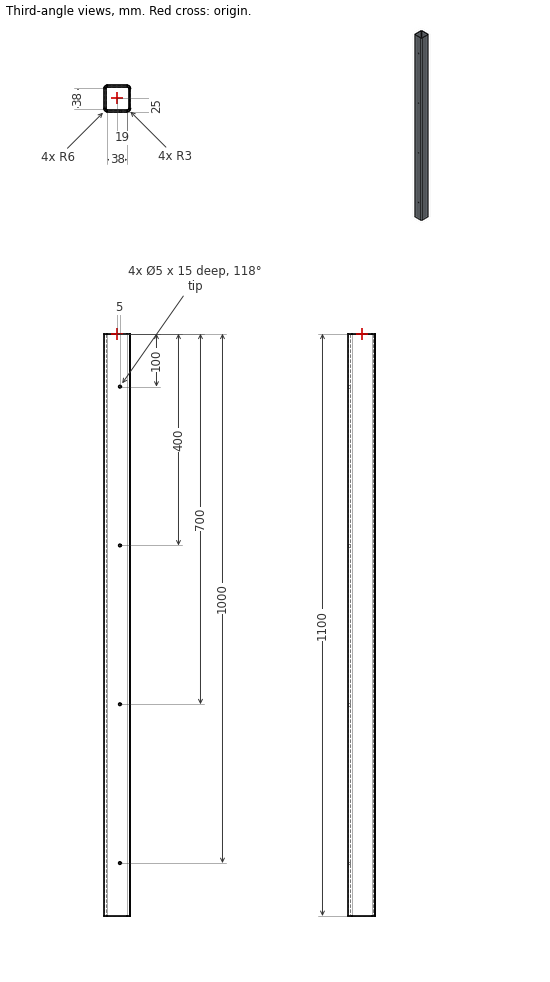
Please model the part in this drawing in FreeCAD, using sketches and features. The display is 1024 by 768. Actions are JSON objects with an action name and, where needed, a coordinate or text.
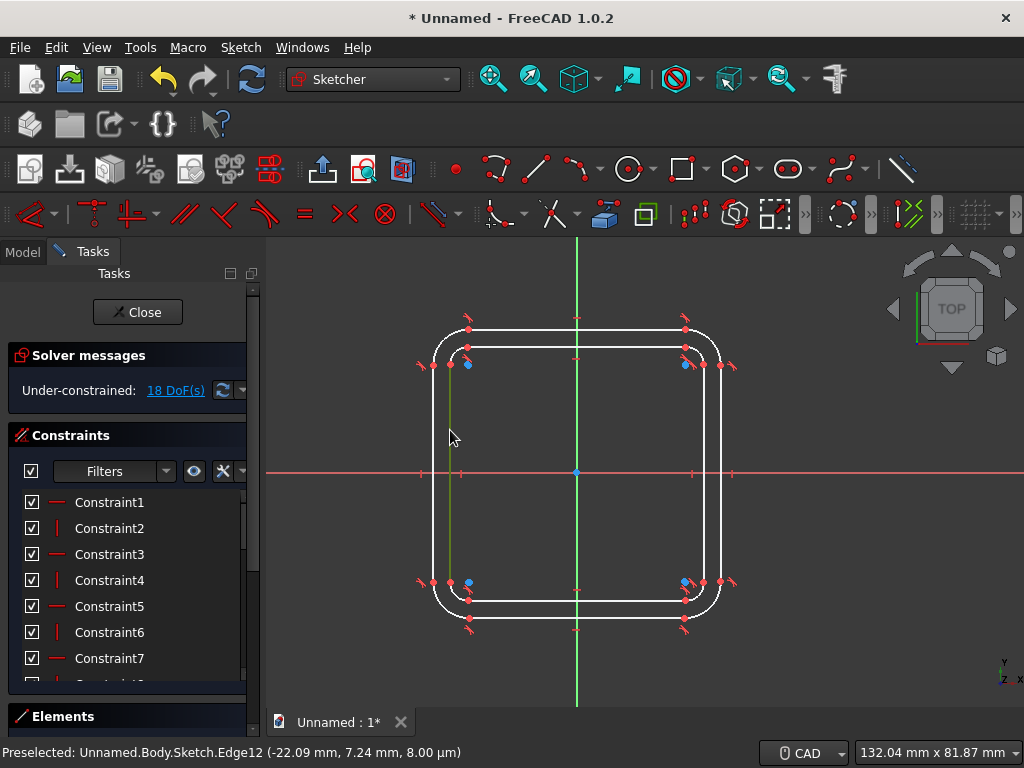
{"action": "left_click", "coordinate": [455, 352]}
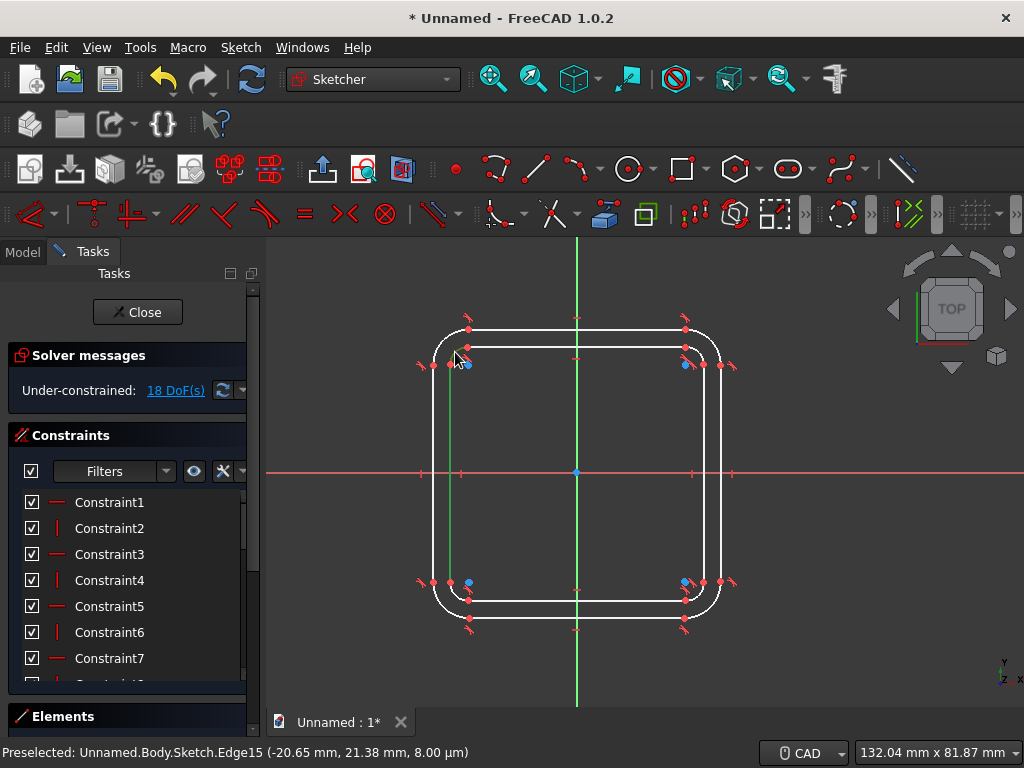
{"action": "key", "text": "t"}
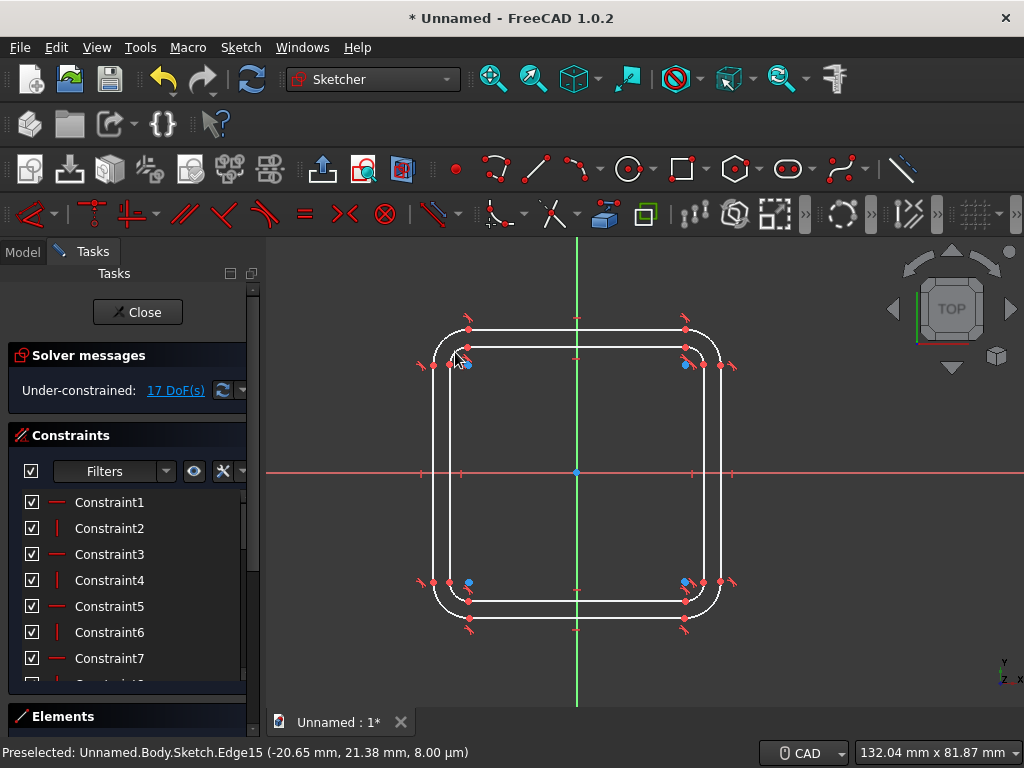
{"action": "left_click", "coordinate": [450, 430]}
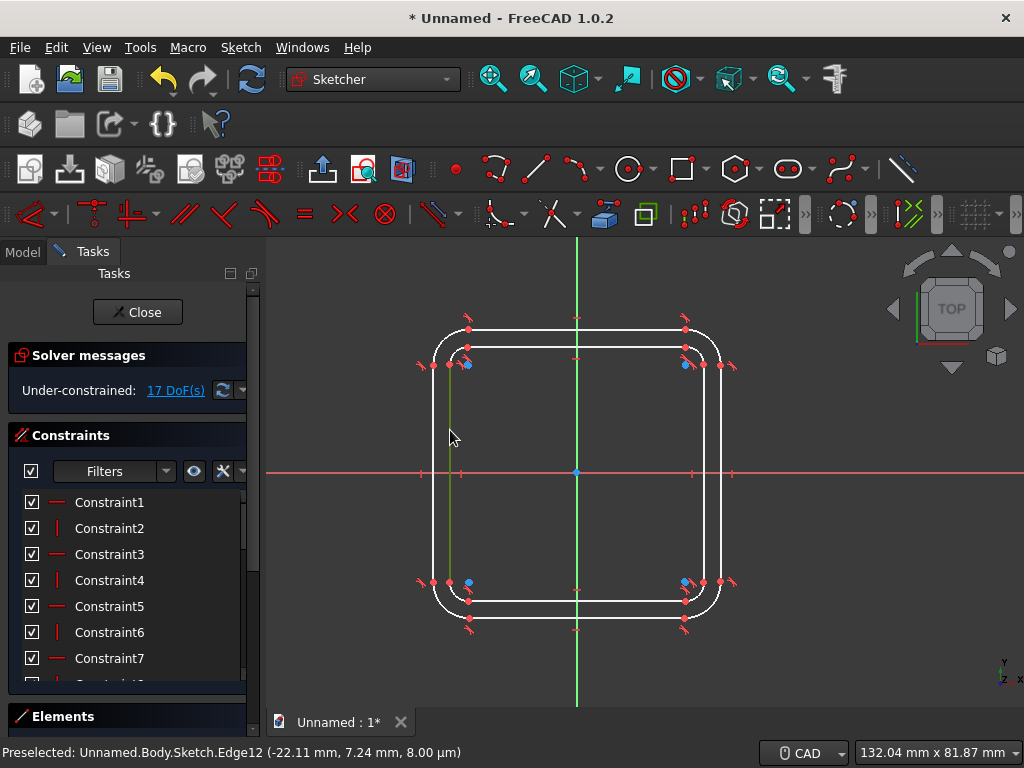
{"action": "left_click", "coordinate": [456, 596]}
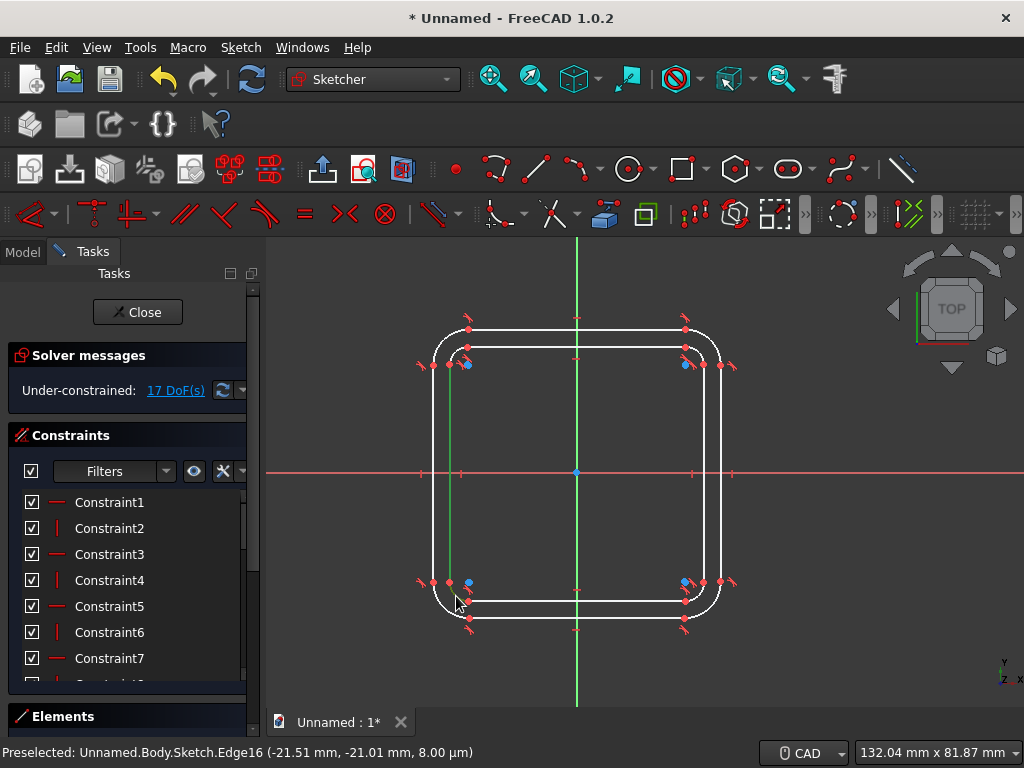
{"action": "key", "text": "t"}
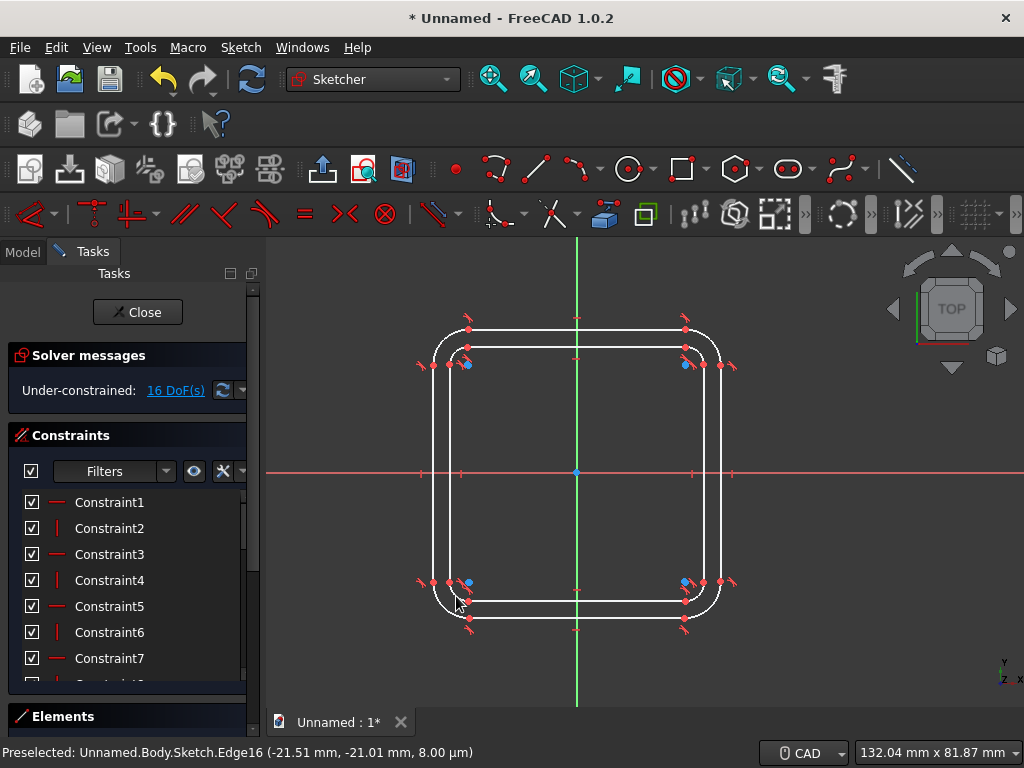
{"action": "left_click", "coordinate": [701, 614]}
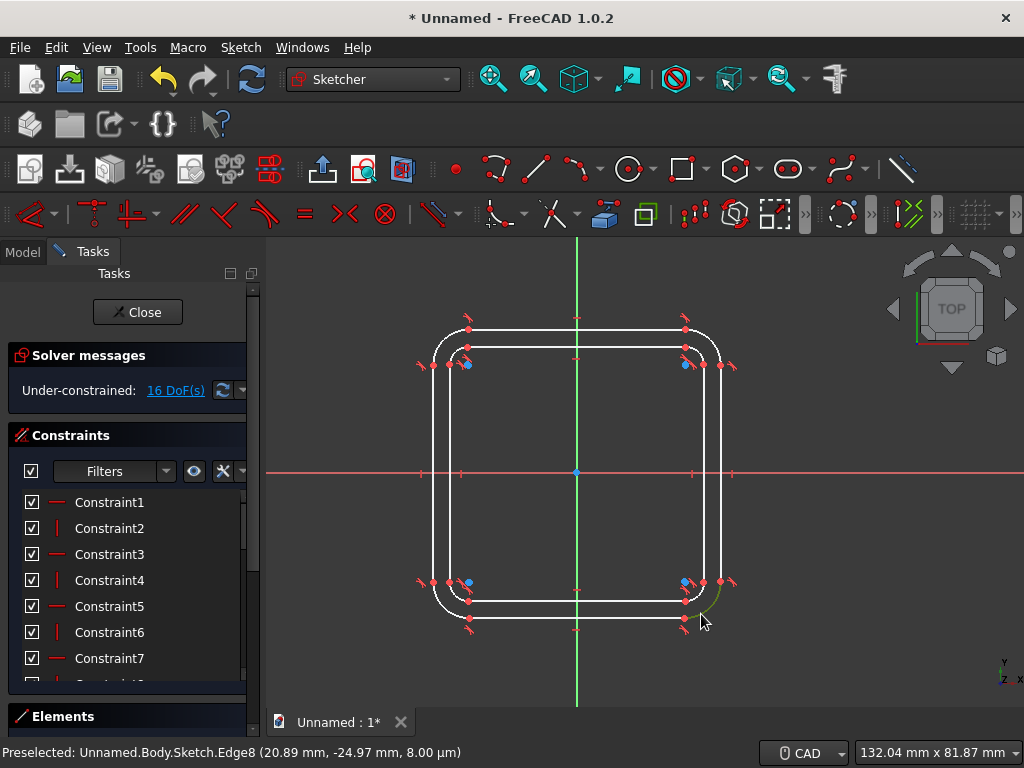
{"action": "left_click", "coordinate": [699, 596]}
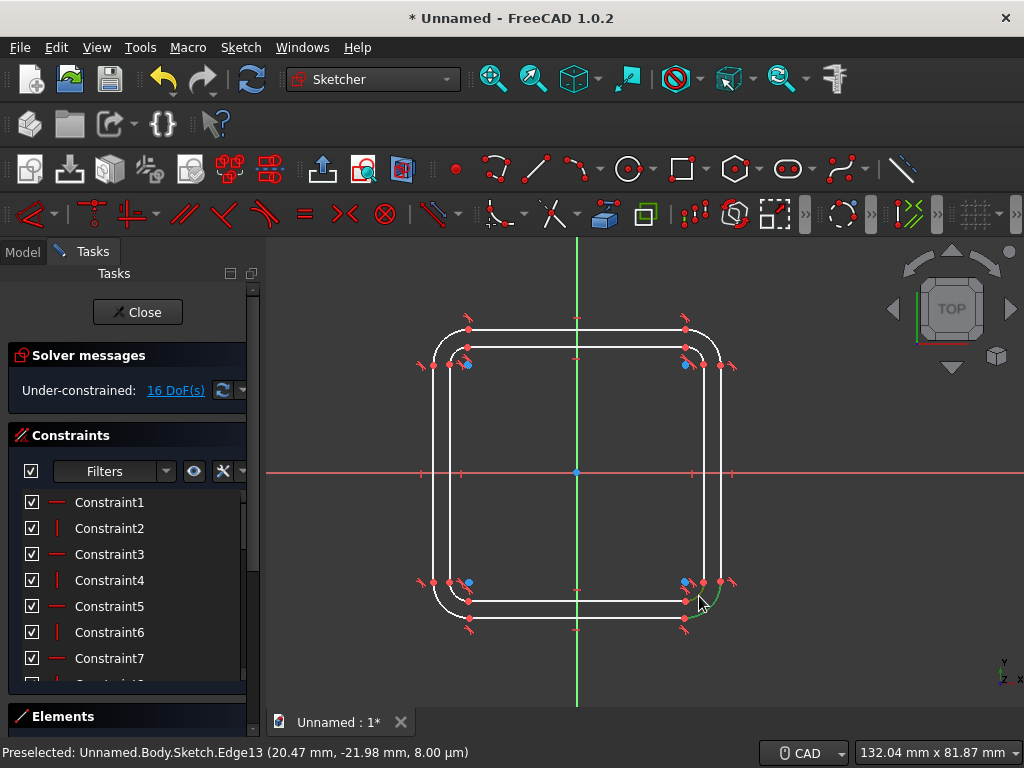
{"action": "key", "text": "c"}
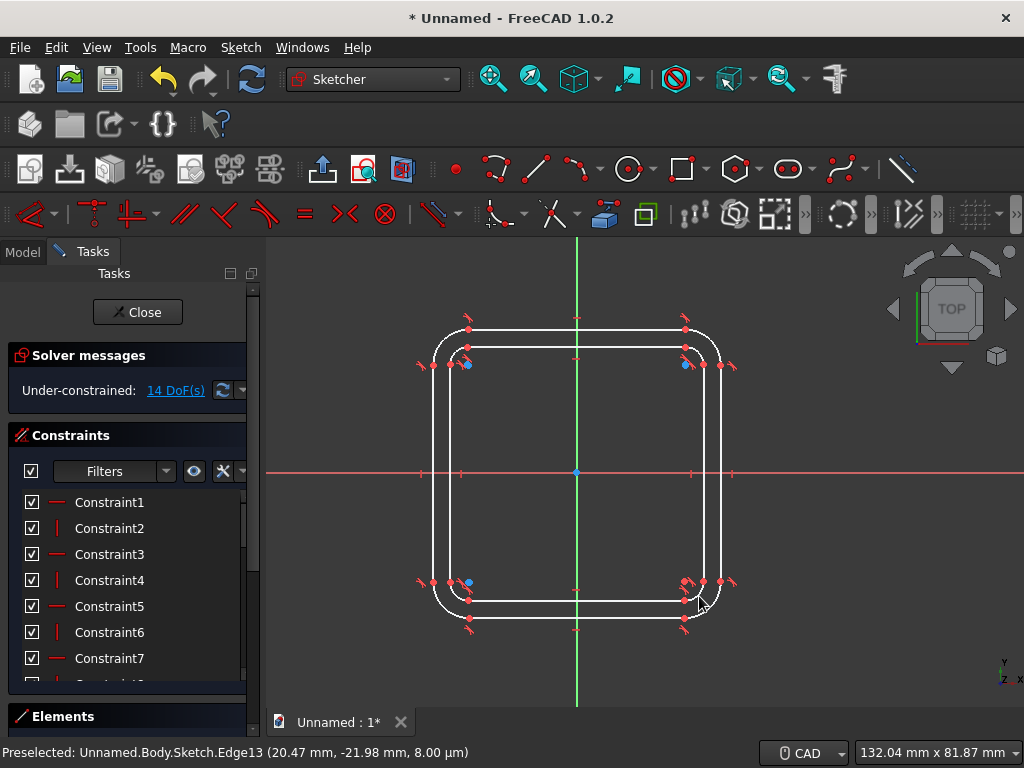
{"action": "left_click", "coordinate": [717, 349]}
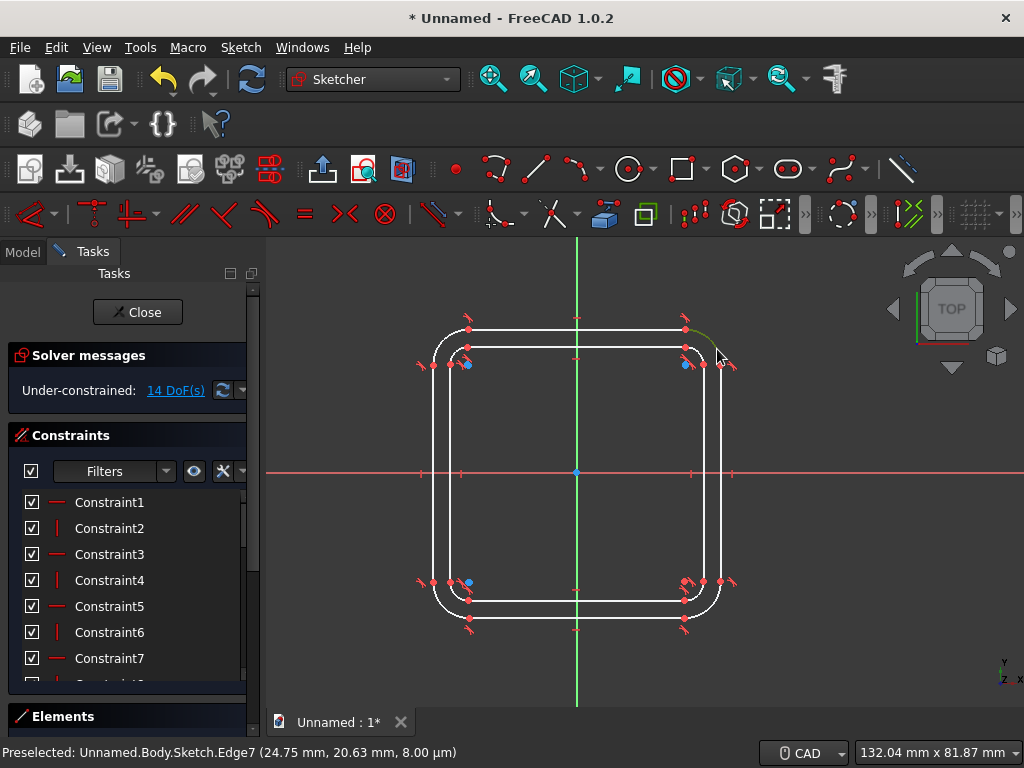
{"action": "left_click", "coordinate": [698, 352]}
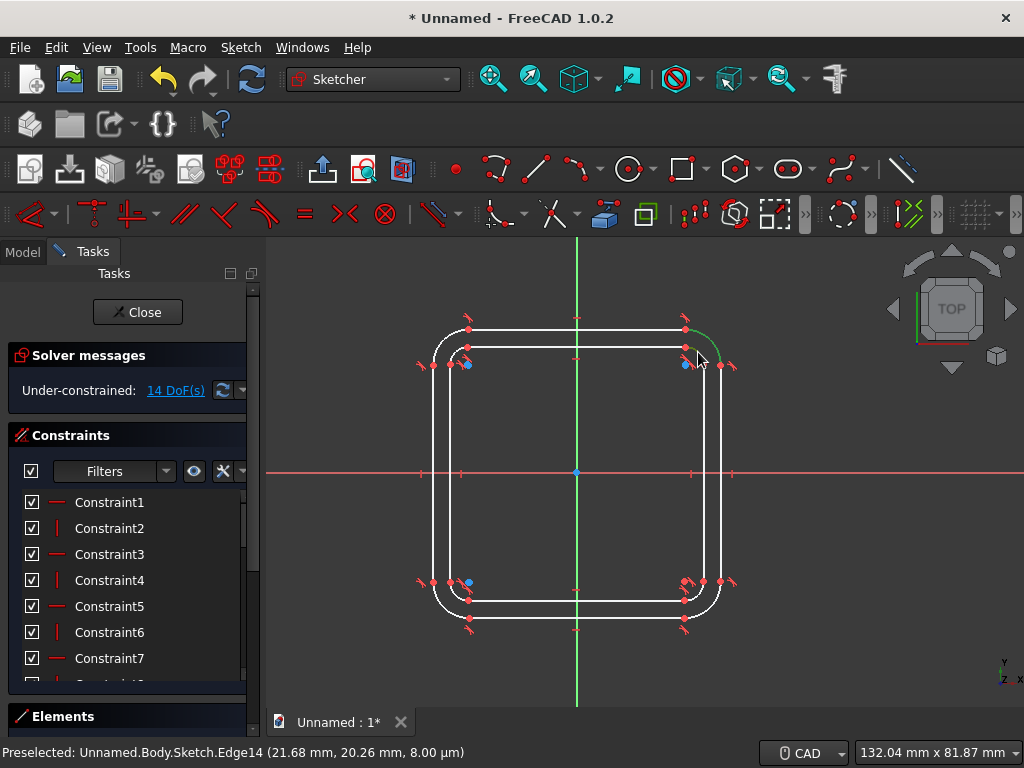
{"action": "key", "text": "c"}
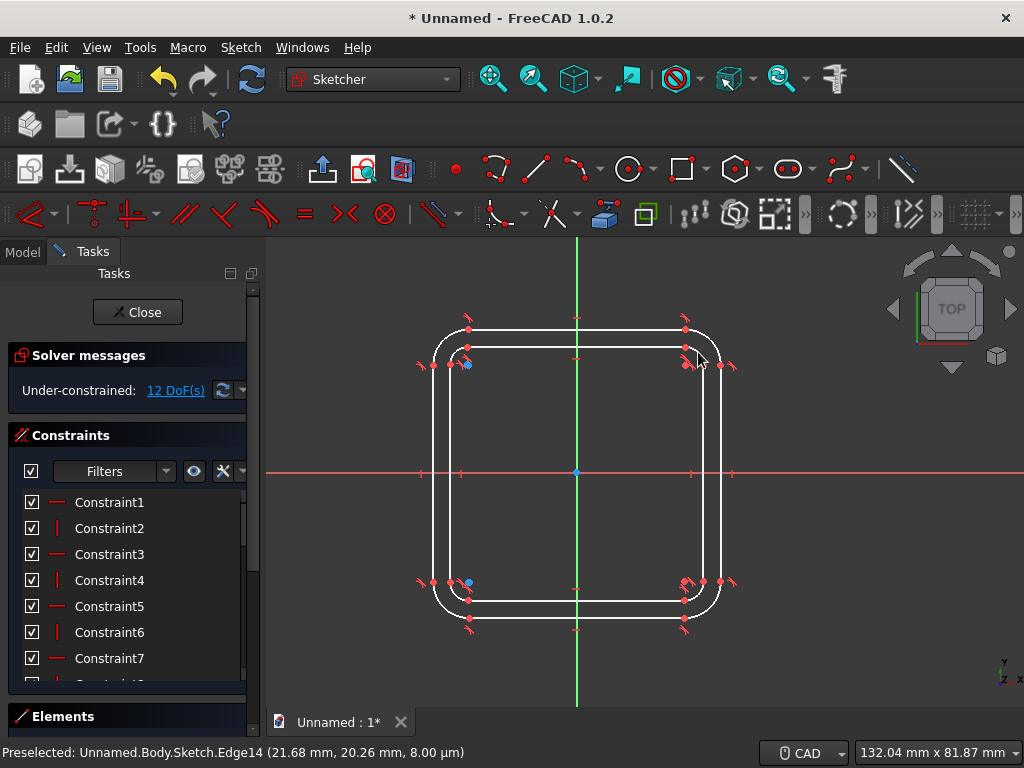
{"action": "left_click", "coordinate": [453, 334]}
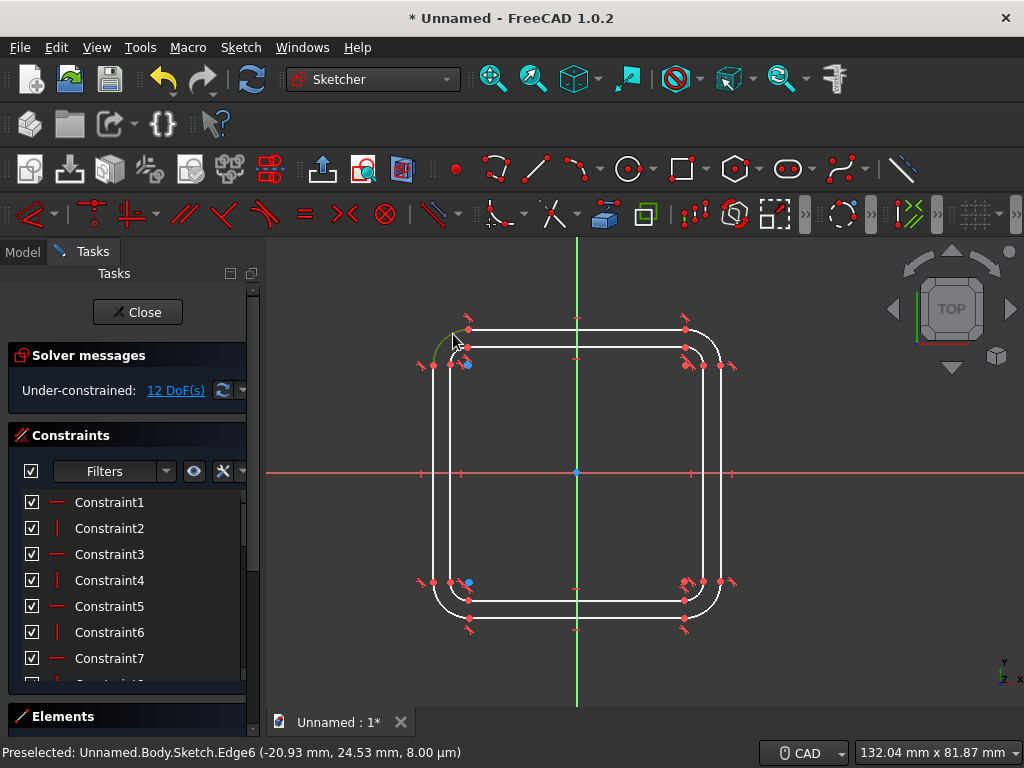
{"action": "left_click", "coordinate": [455, 352]}